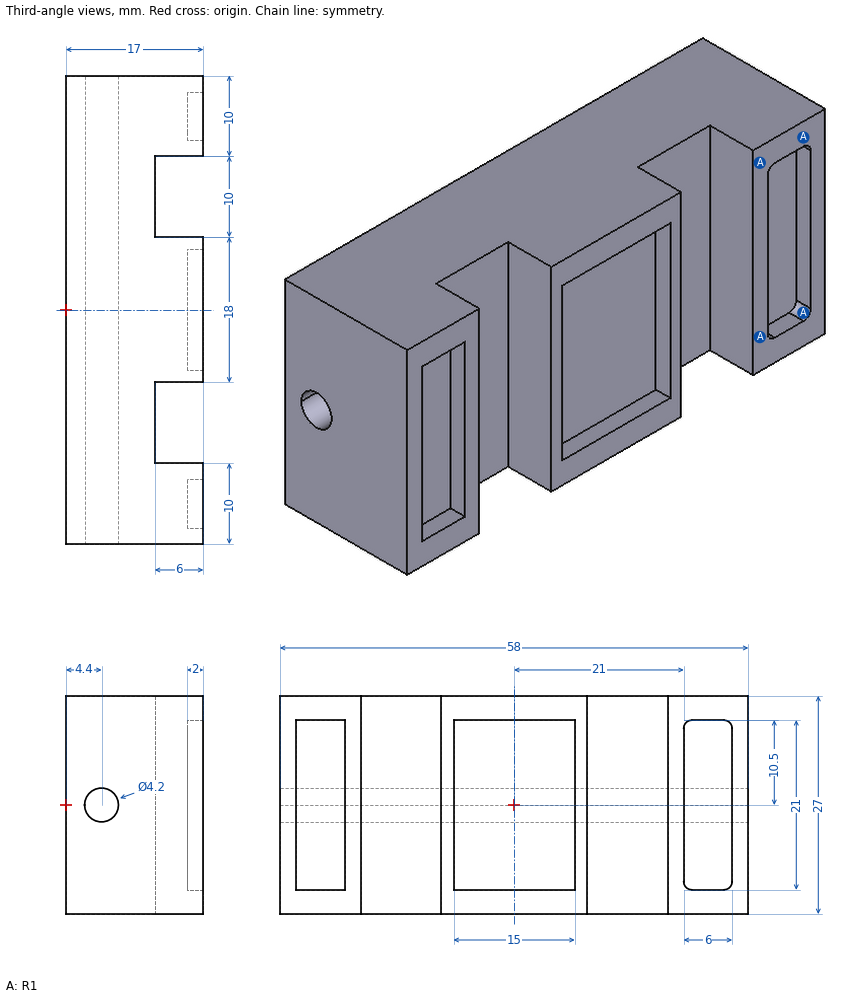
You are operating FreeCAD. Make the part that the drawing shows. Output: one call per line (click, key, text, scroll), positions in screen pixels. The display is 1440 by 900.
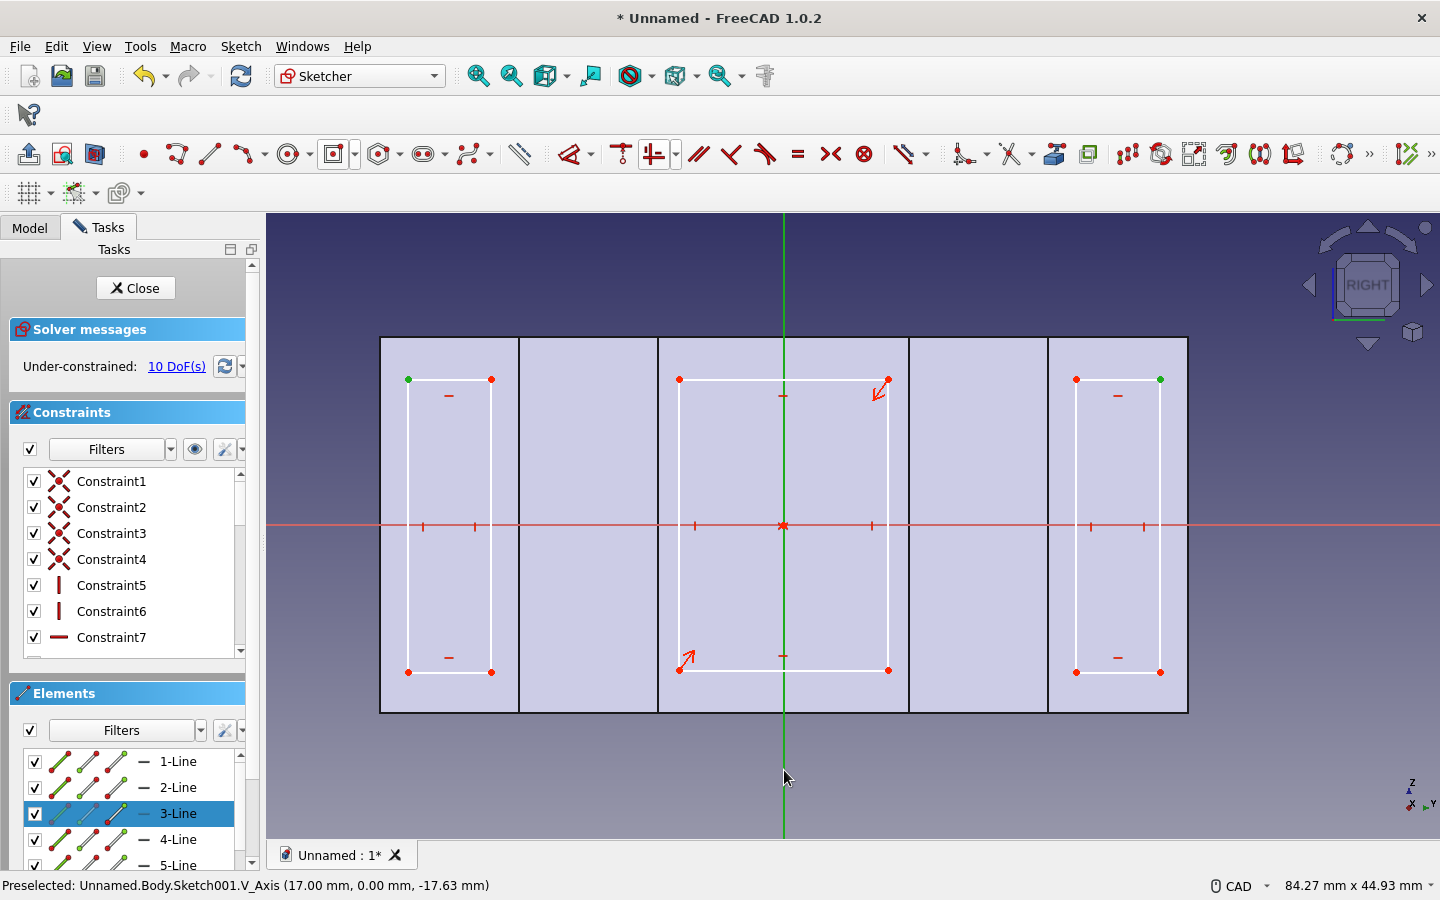
key(s)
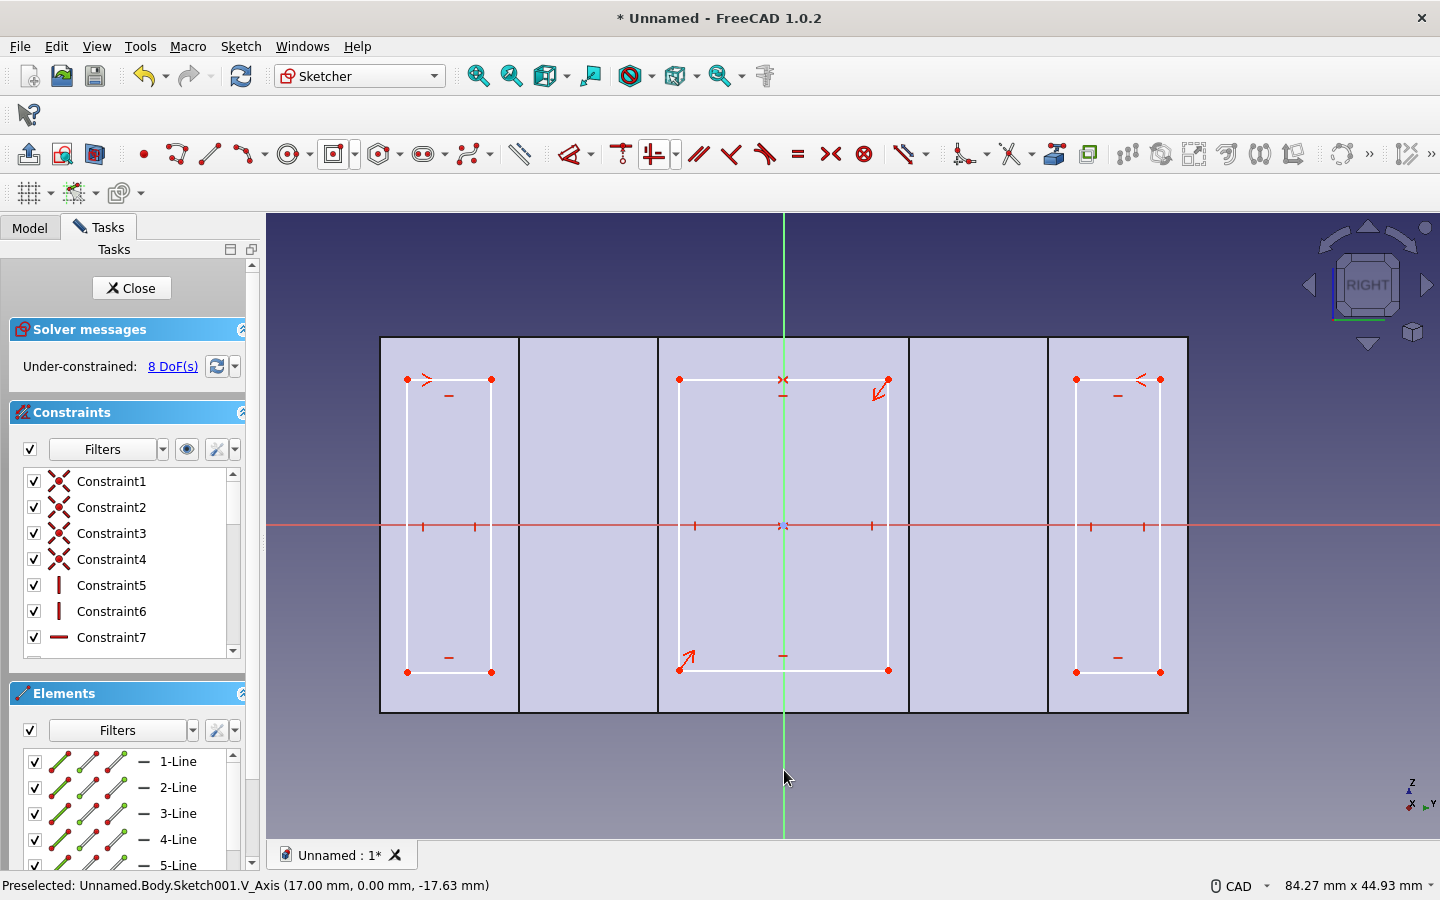
click(1076, 673)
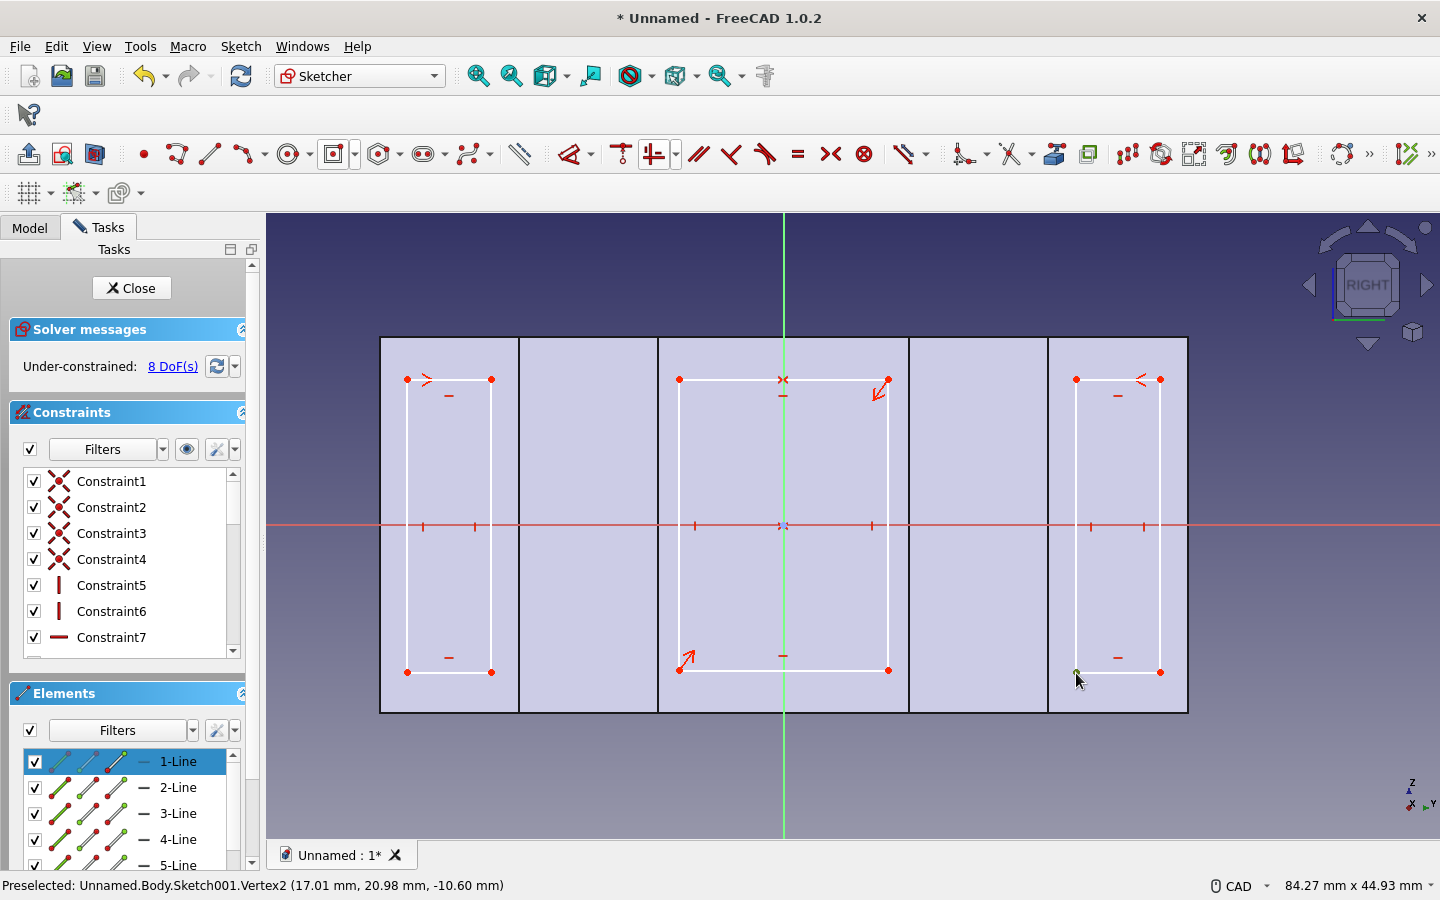
click(491, 673)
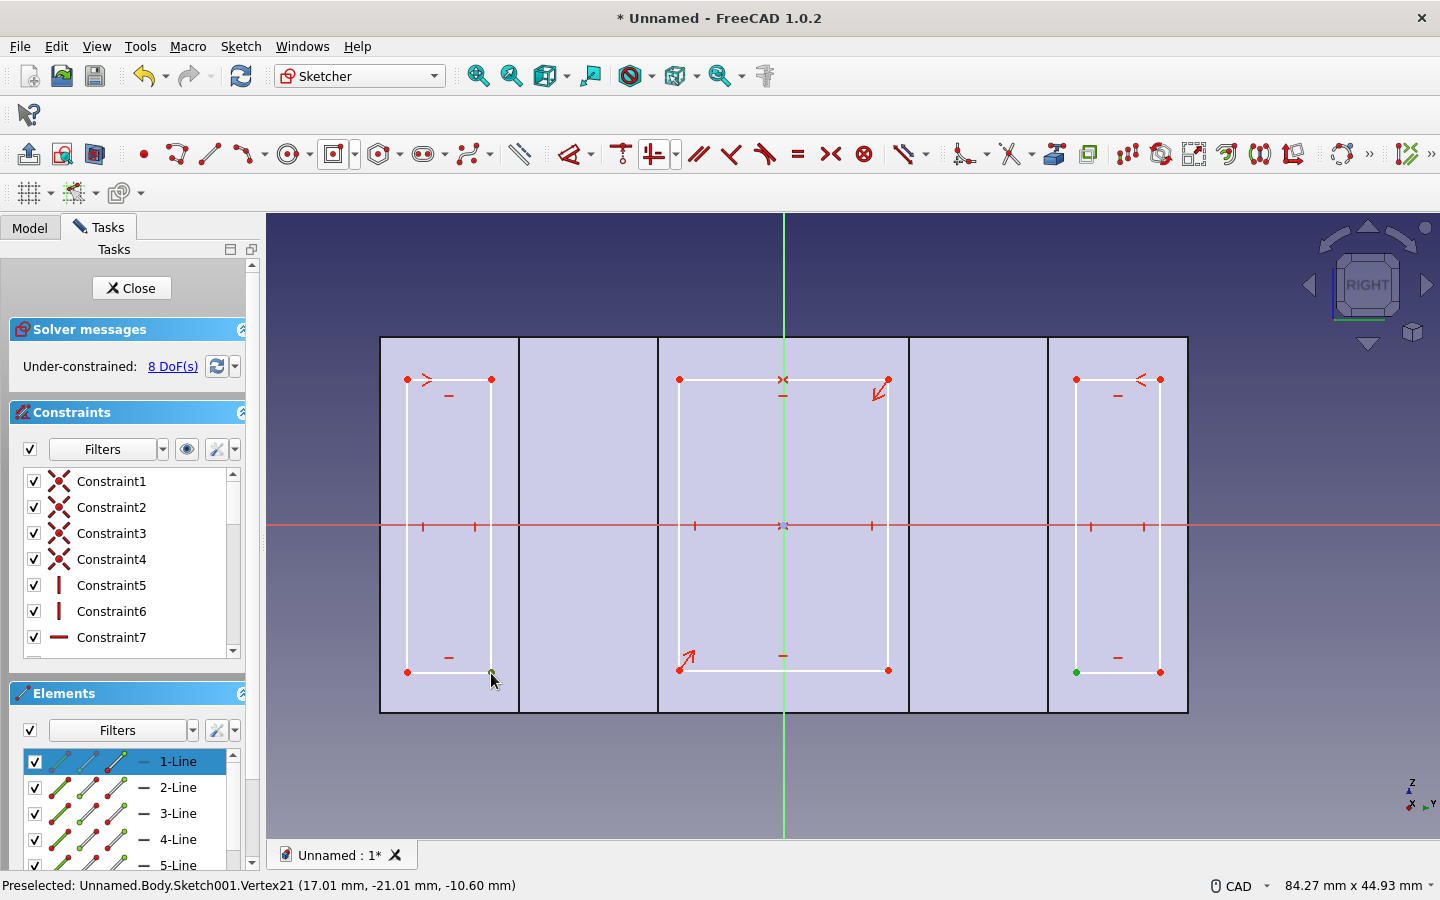
click(784, 770)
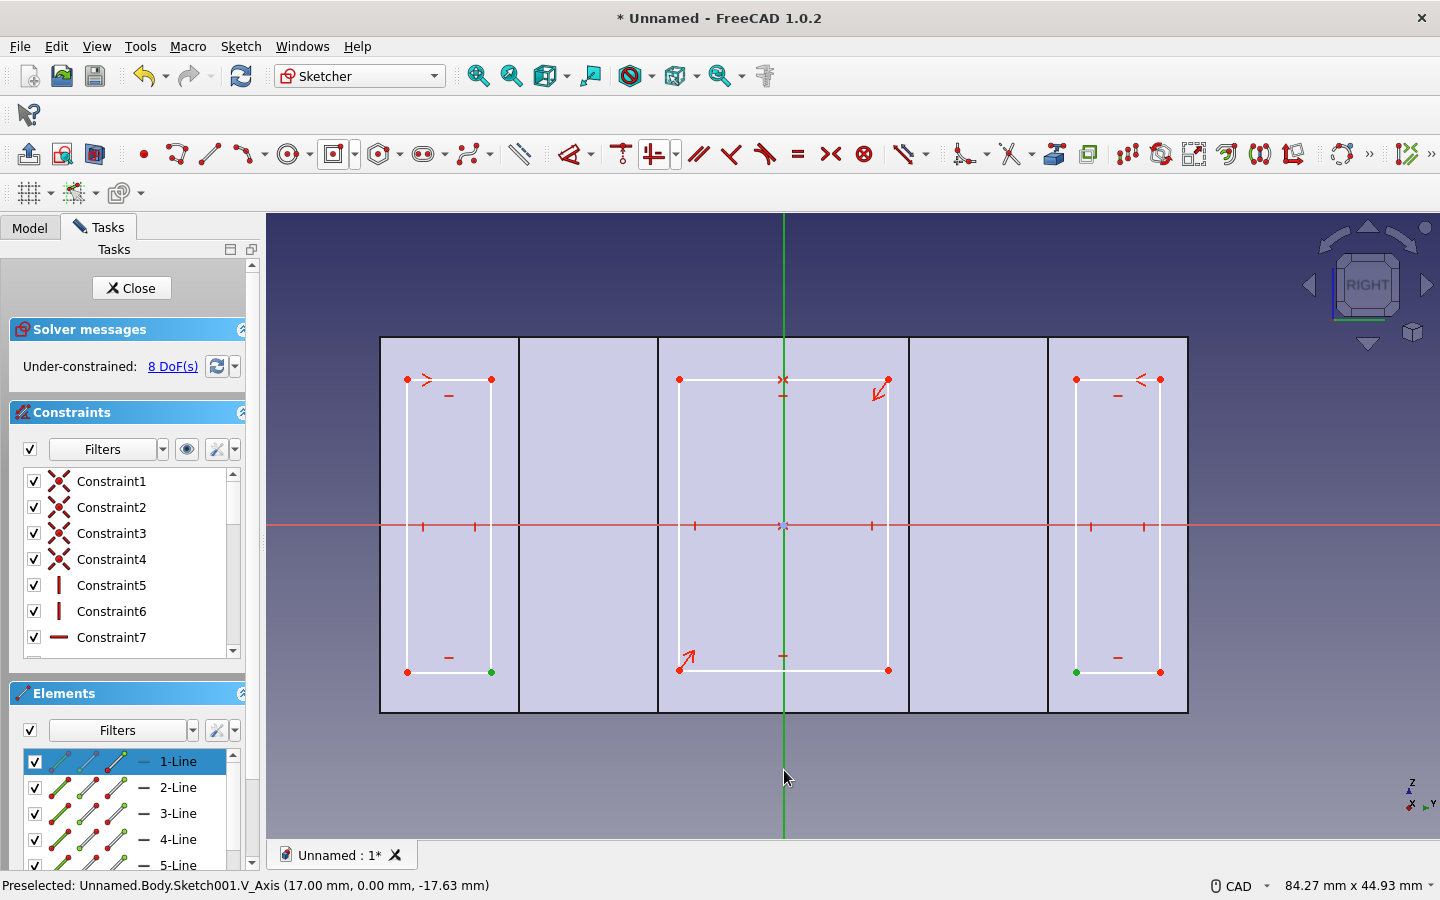
click(831, 154)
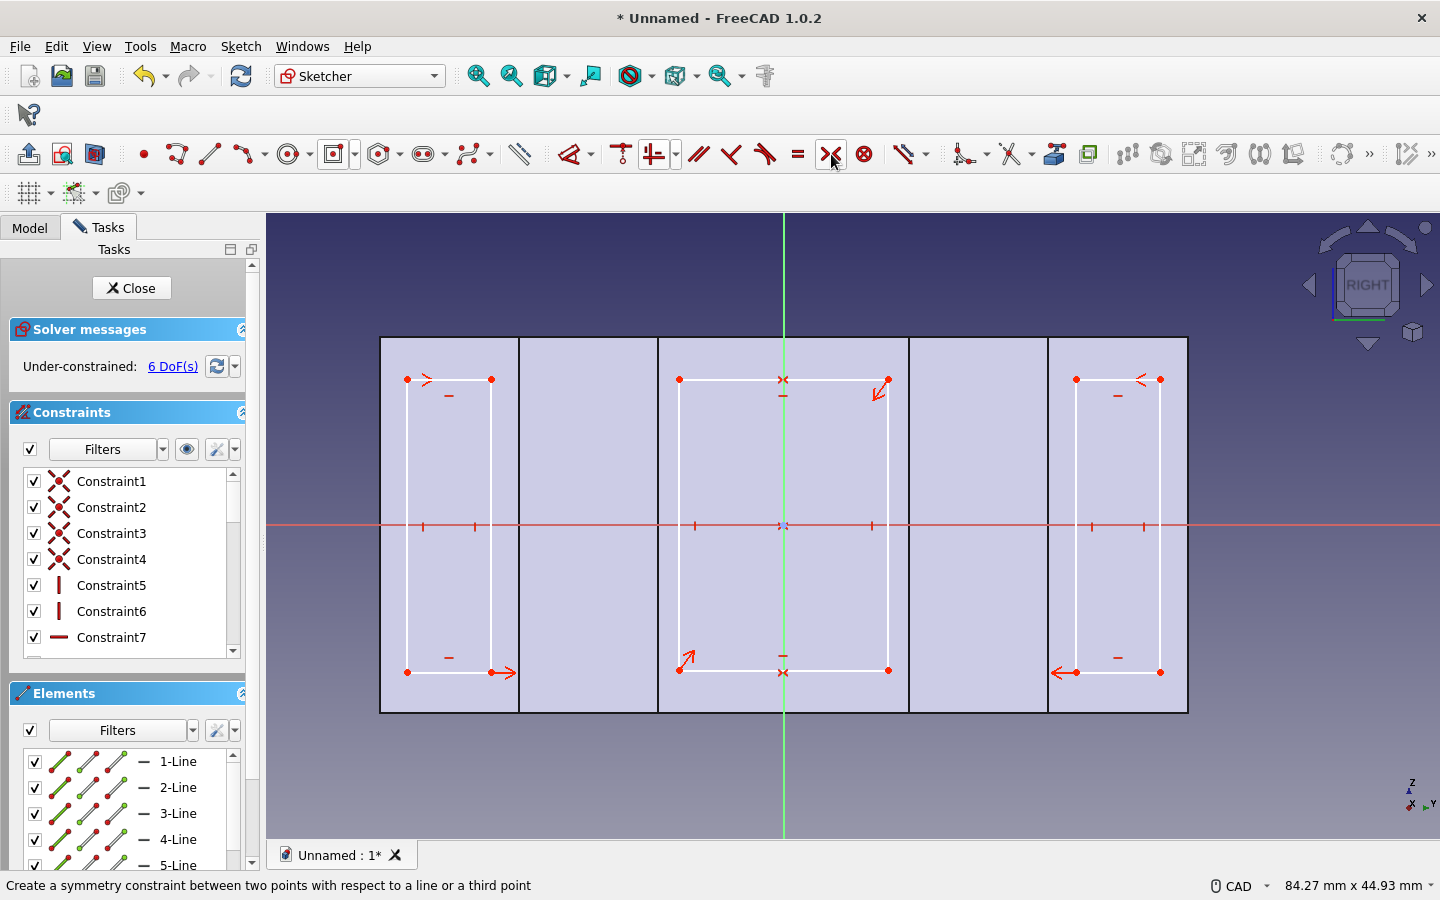
key(d)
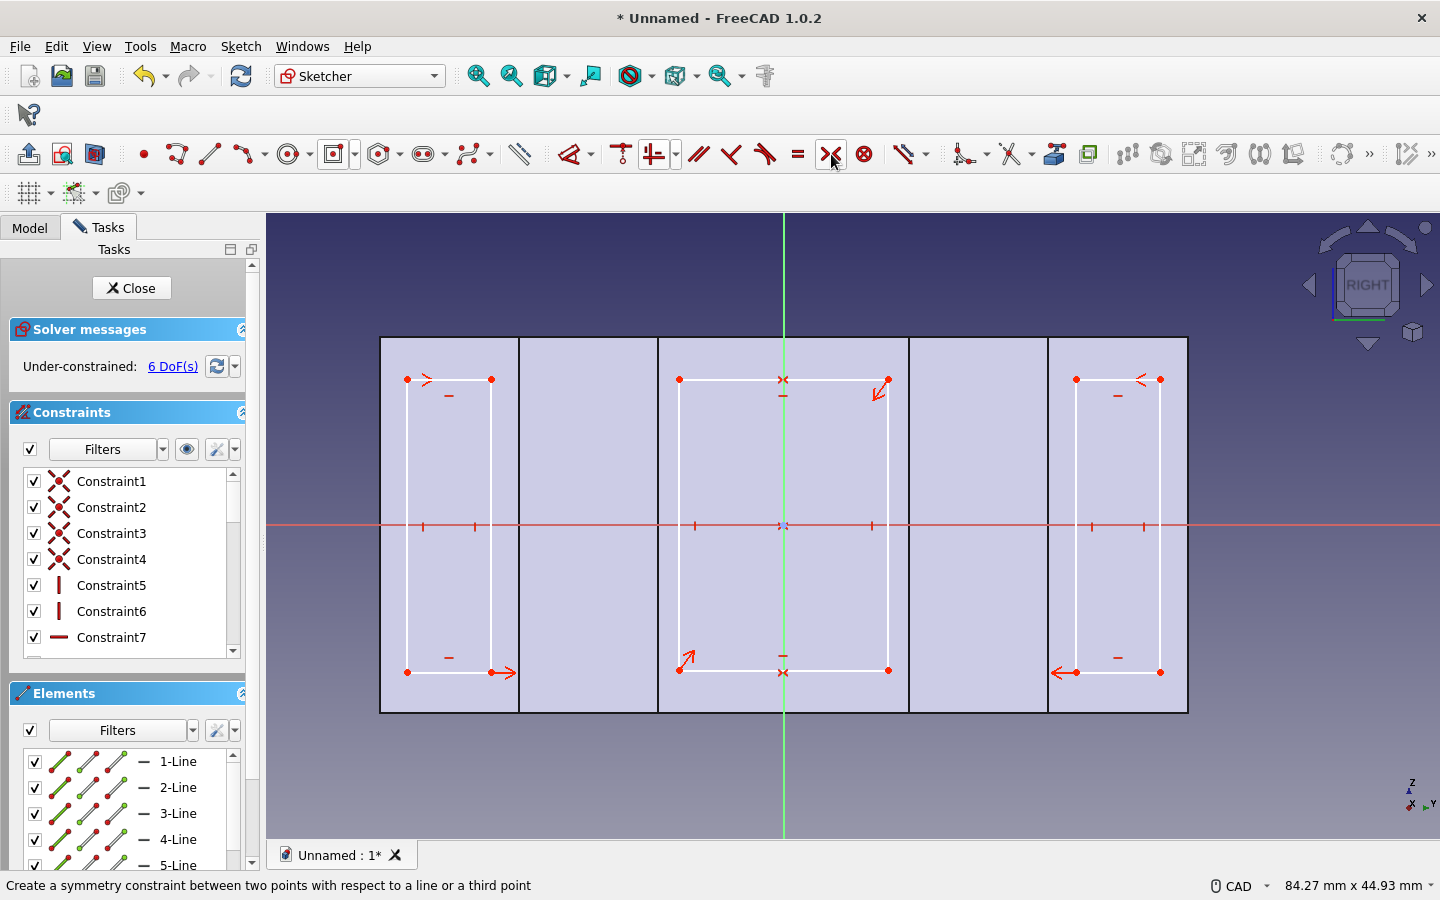
click(1101, 673)
click(1118, 707)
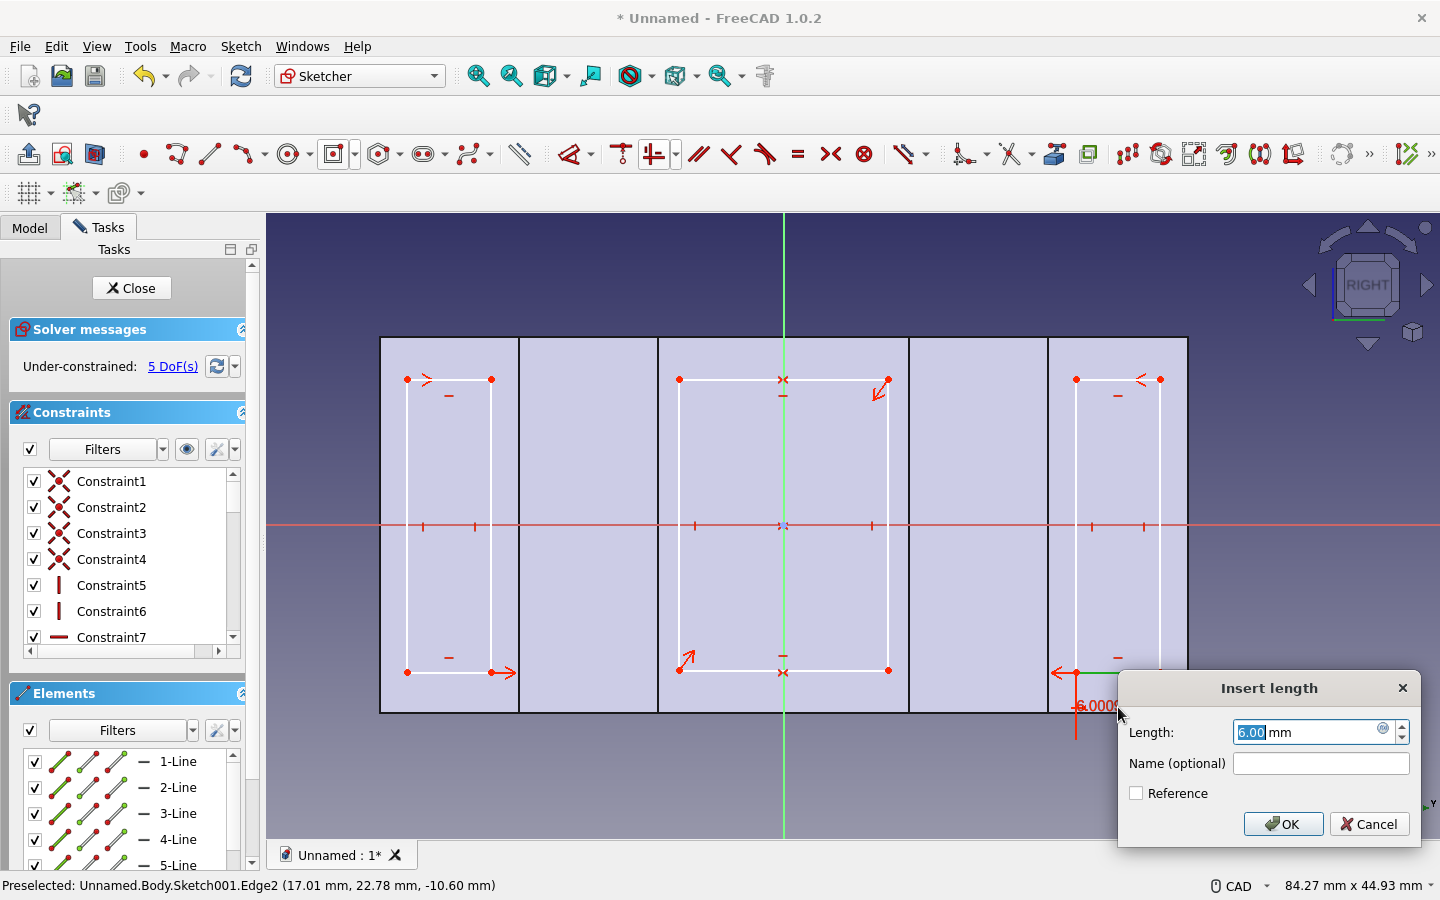
text(6)
key(Return)